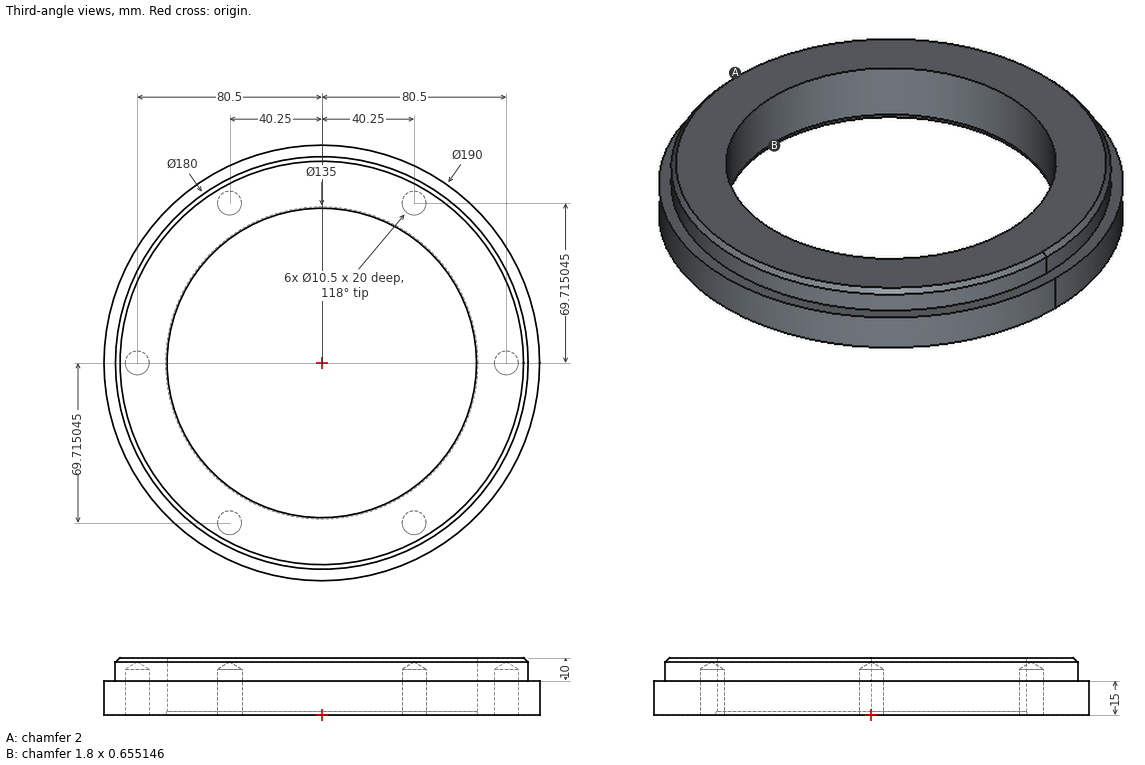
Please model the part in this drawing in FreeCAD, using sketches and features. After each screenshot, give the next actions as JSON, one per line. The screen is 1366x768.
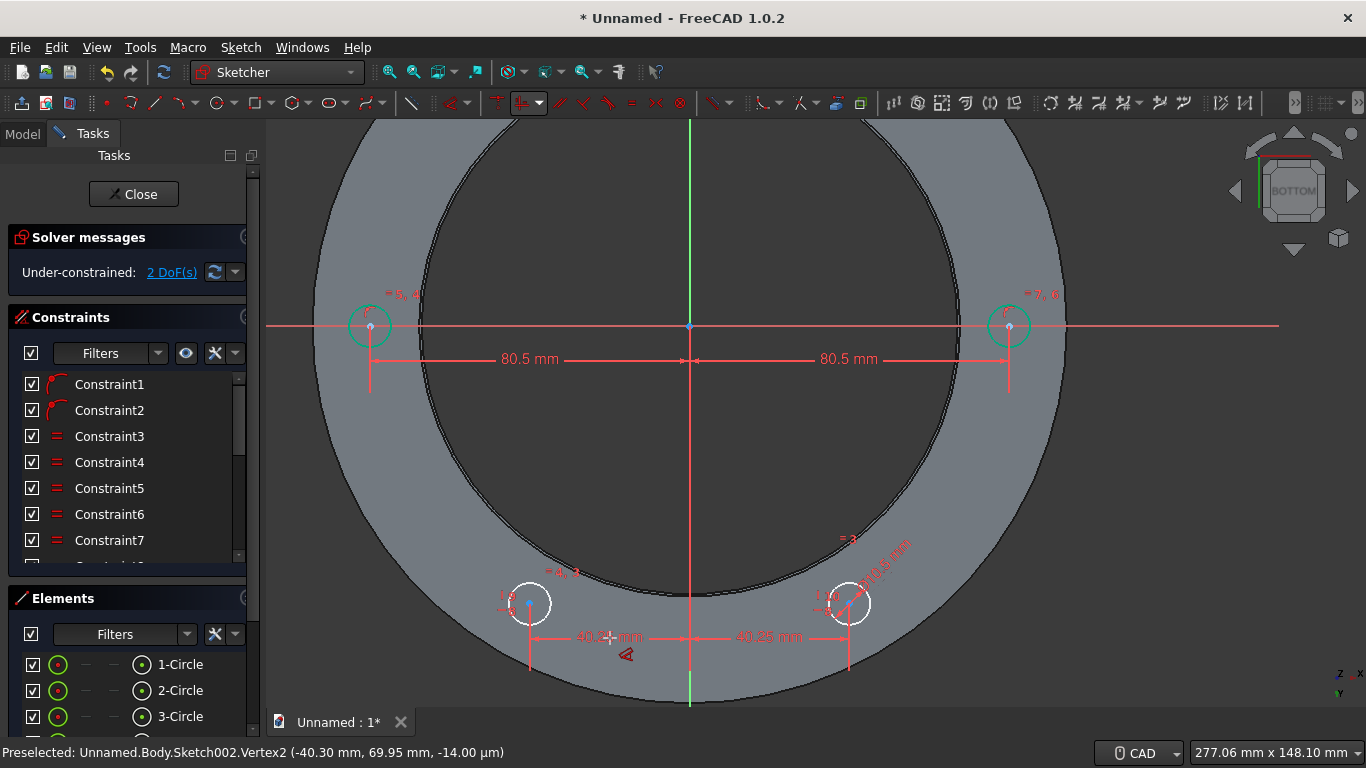
{"action": "left_click", "coordinate": [849, 604]}
{"action": "left_click", "coordinate": [883, 465]}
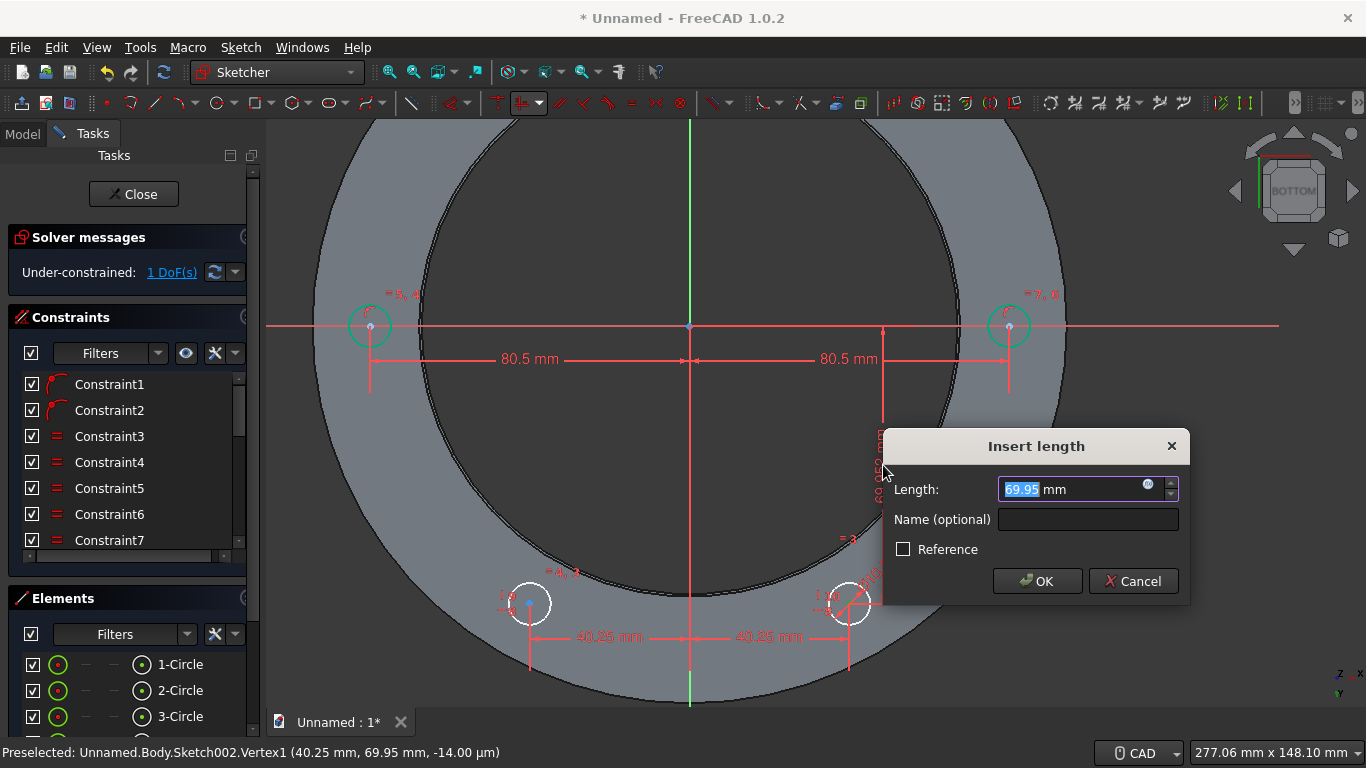
{"action": "type", "text": "69.715045"}
{"action": "key", "text": "Return"}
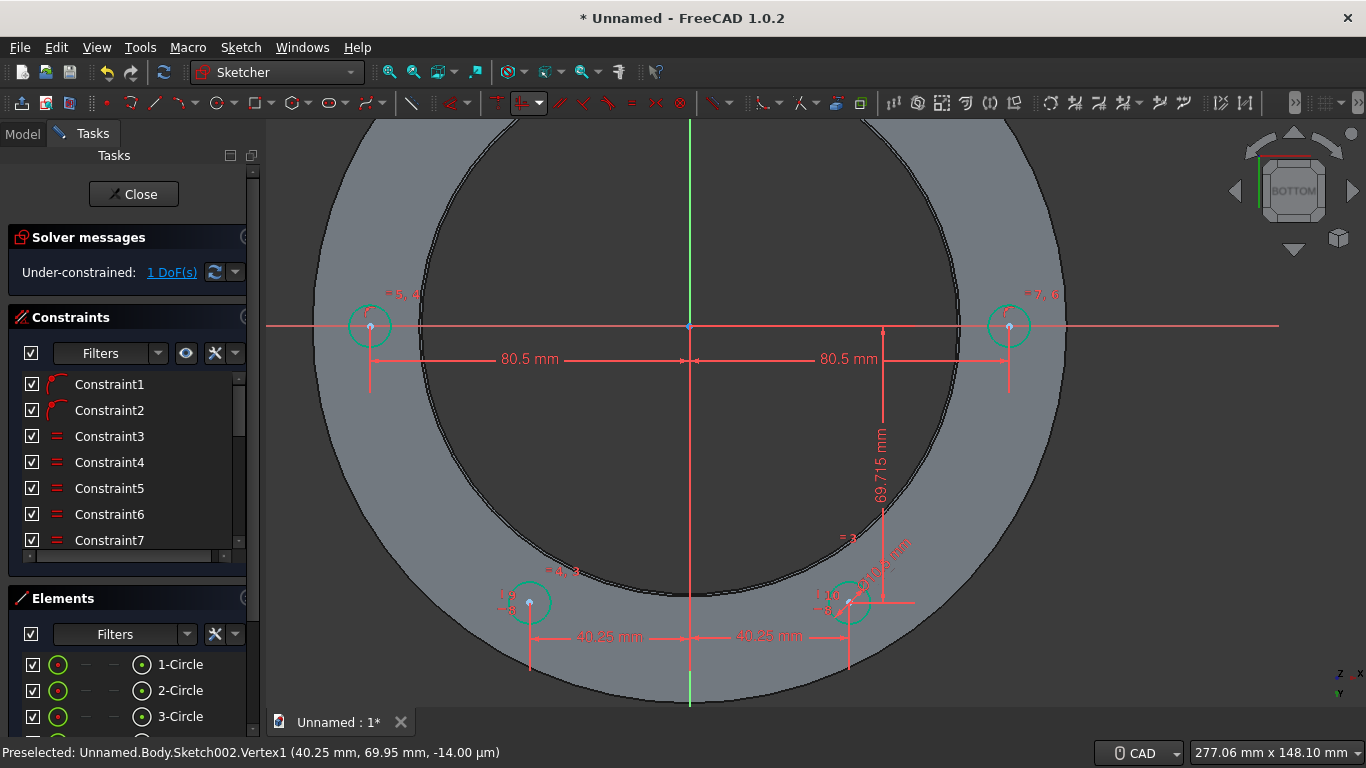
{"action": "scroll", "coordinate": [865, 590], "scroll_direction": "down", "scroll_amount": 2}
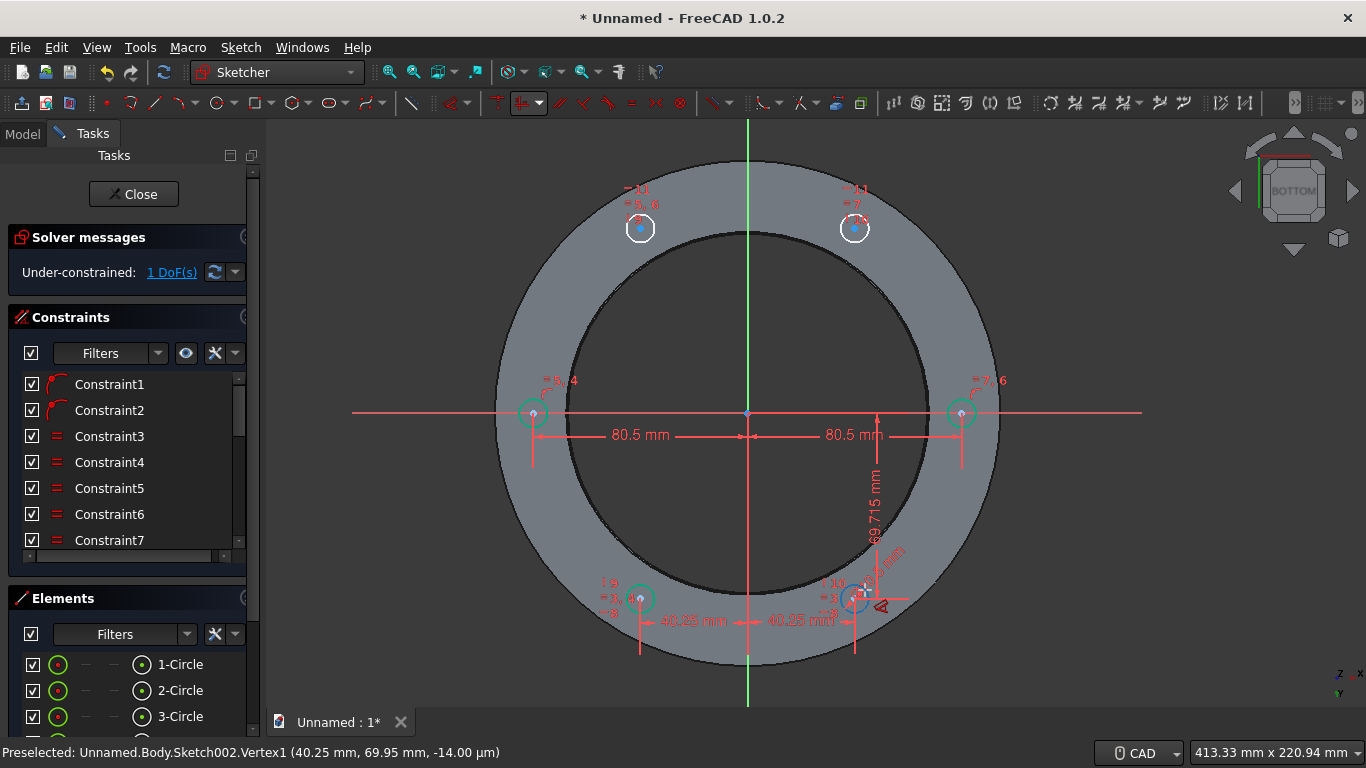
{"action": "left_click", "coordinate": [640, 229]}
{"action": "left_click", "coordinate": [606, 321]}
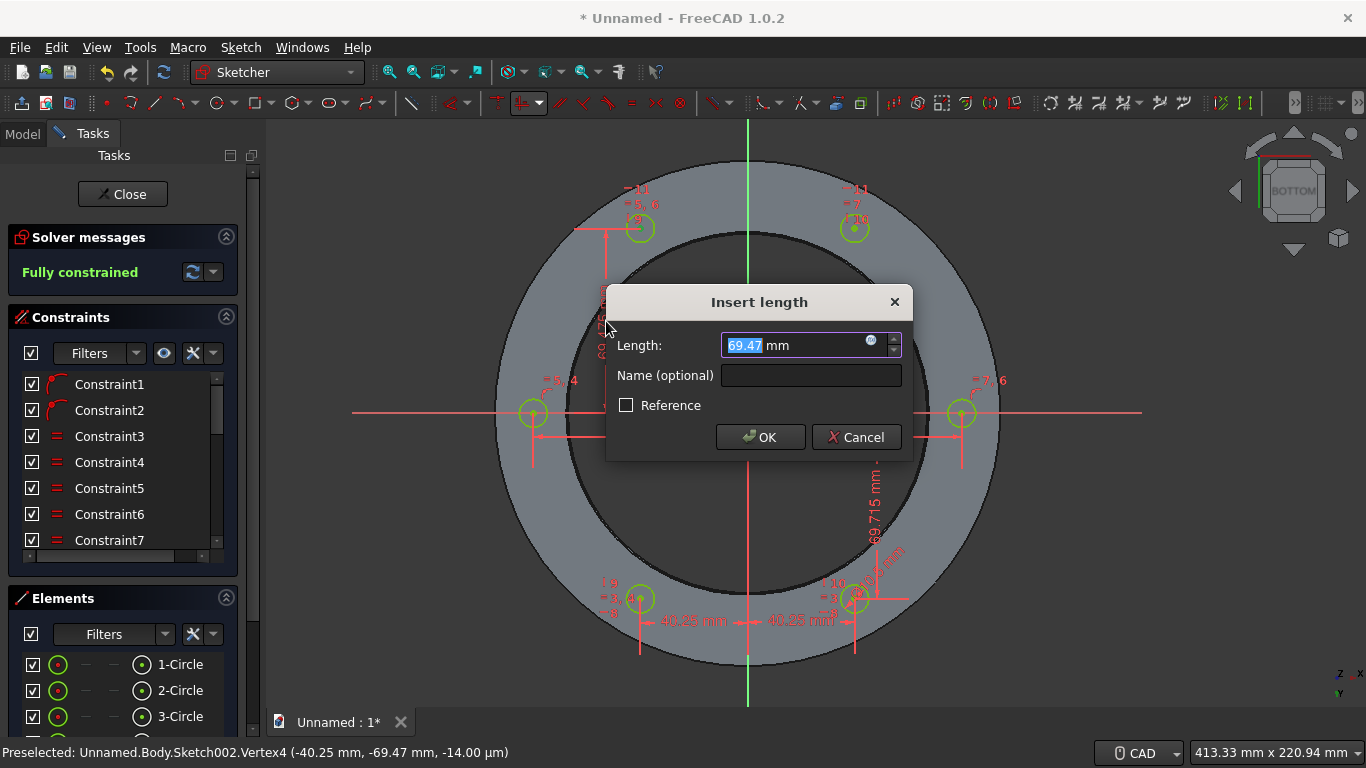
{"action": "type", "text": "69.715045"}
{"action": "key", "text": "Return"}
{"action": "key", "text": "Escape"}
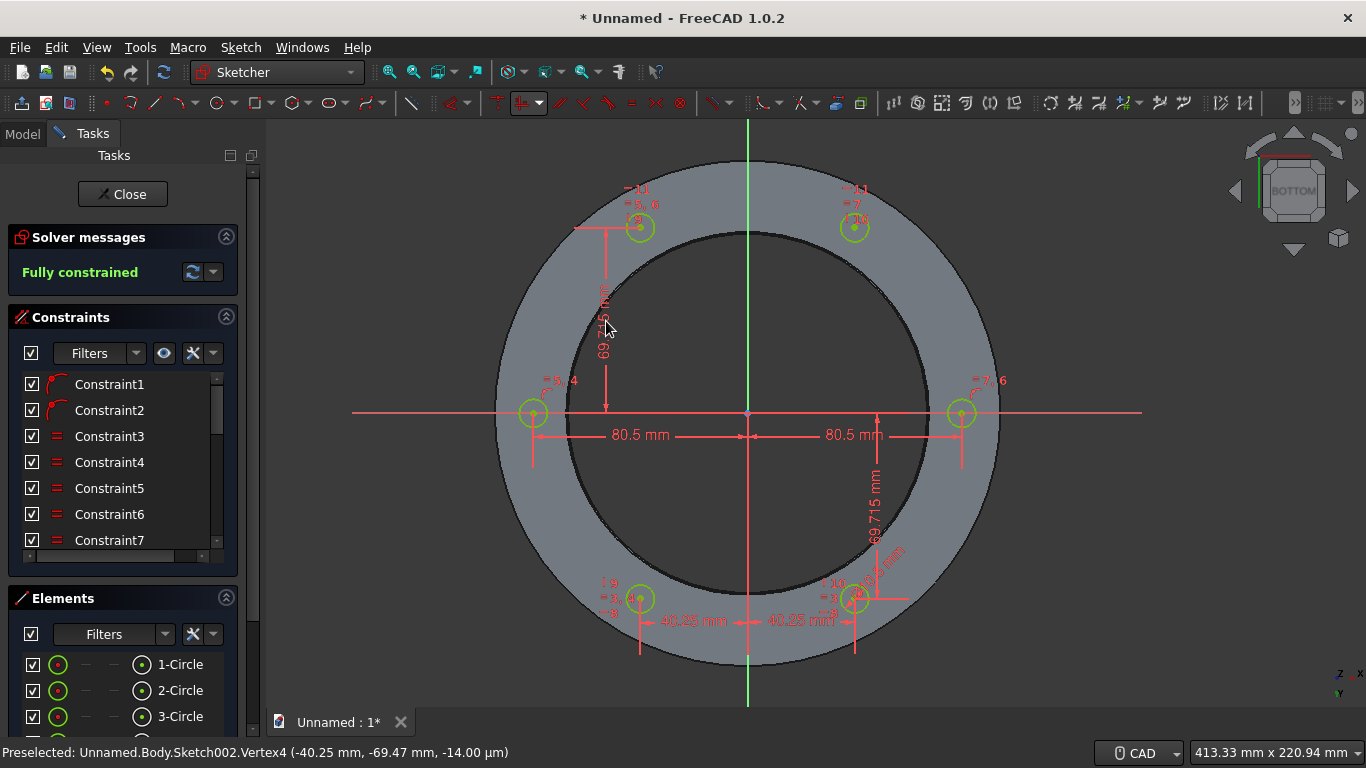
{"action": "left_click", "coordinate": [123, 194]}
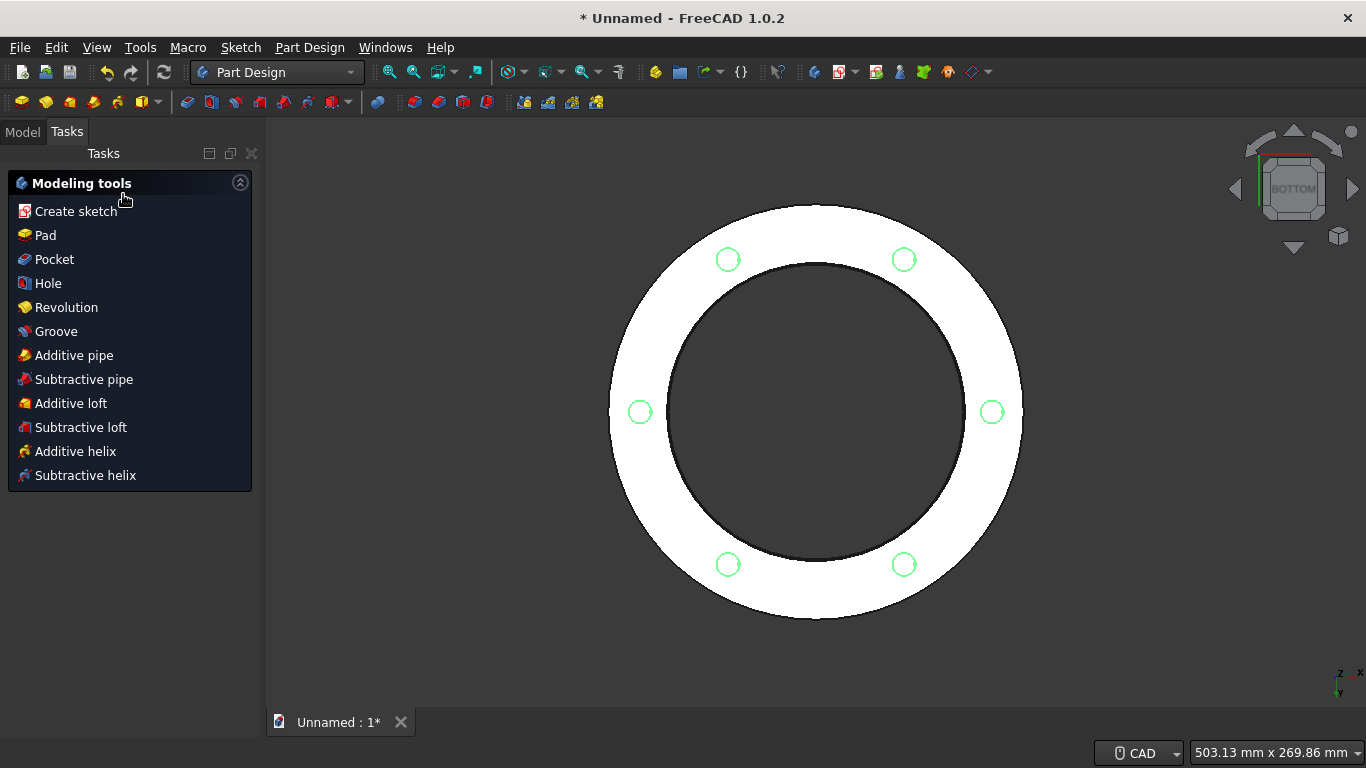
{"action": "left_click", "coordinate": [212, 102]}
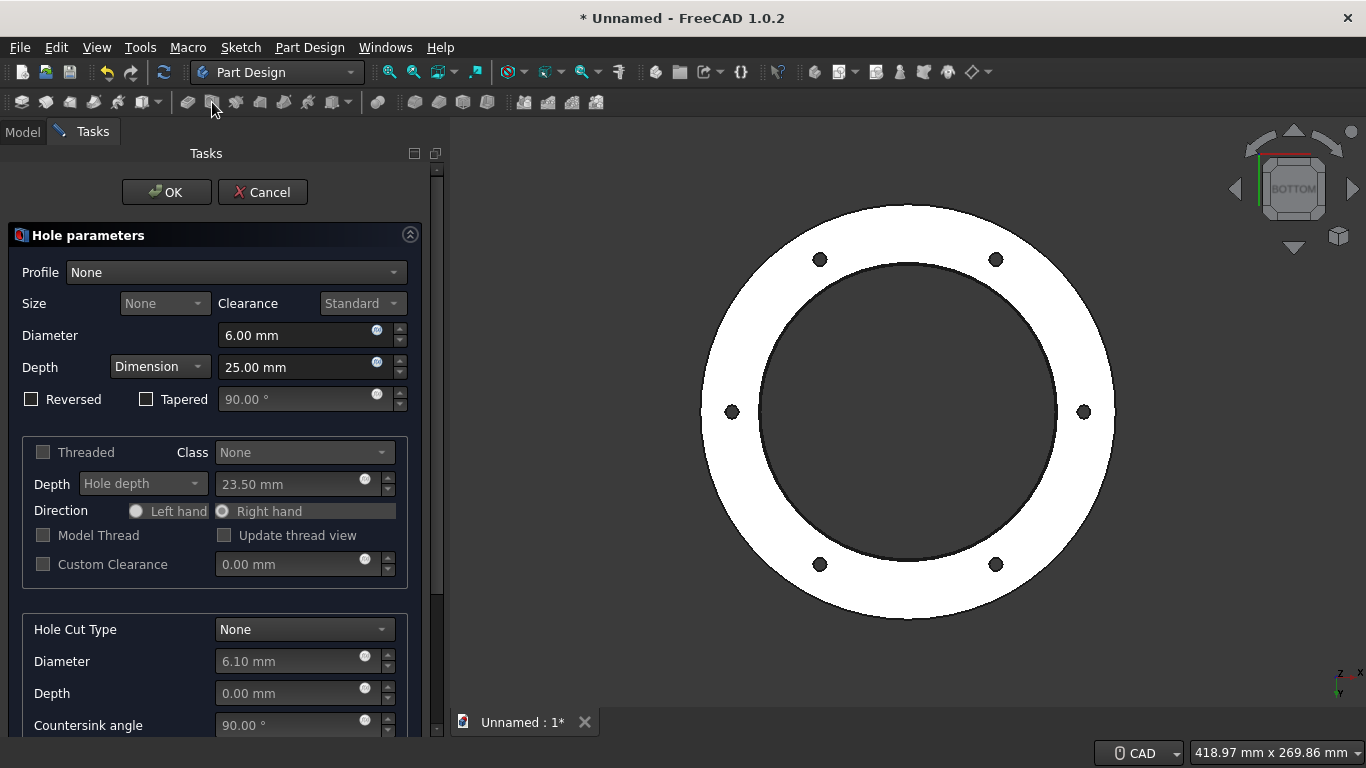
{"action": "triple_click", "coordinate": [305, 335]}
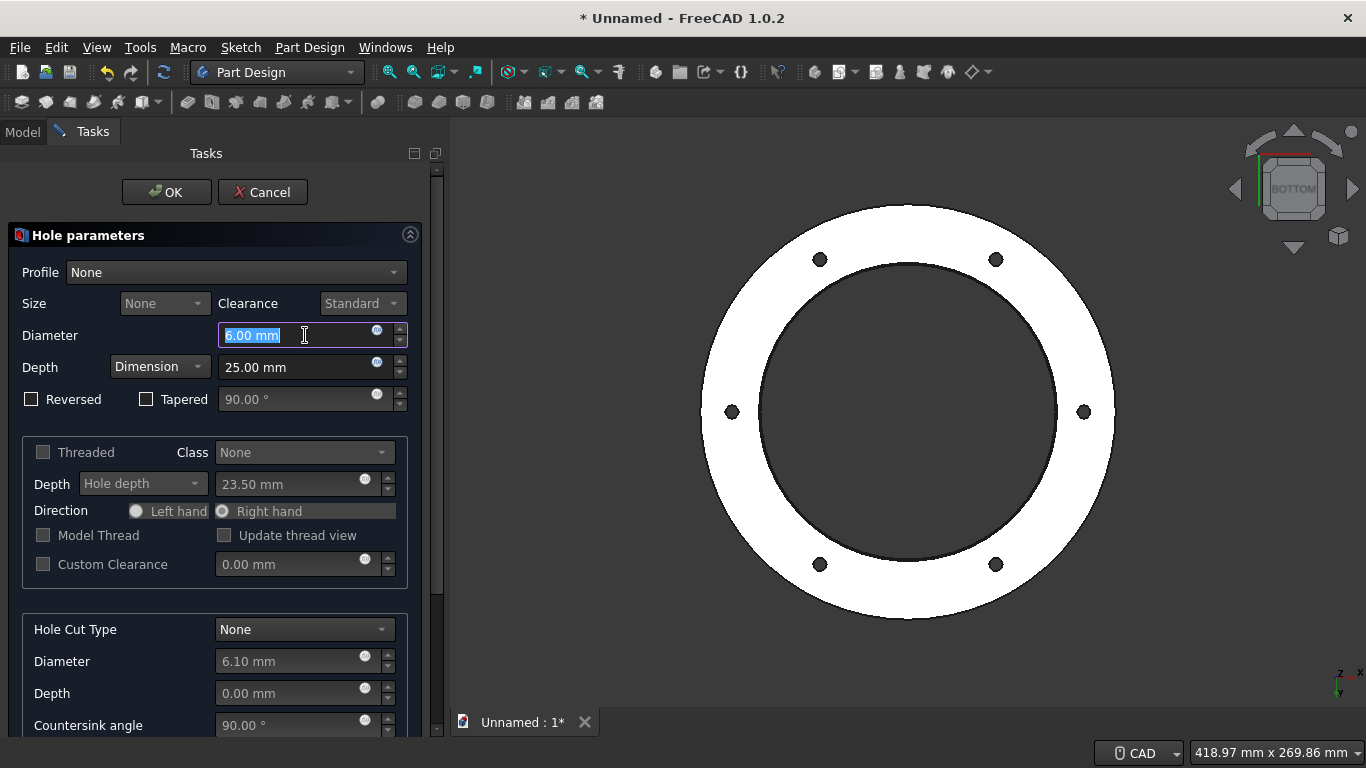
{"action": "type", "text": "10.5"}
{"action": "key", "text": "Tab"}